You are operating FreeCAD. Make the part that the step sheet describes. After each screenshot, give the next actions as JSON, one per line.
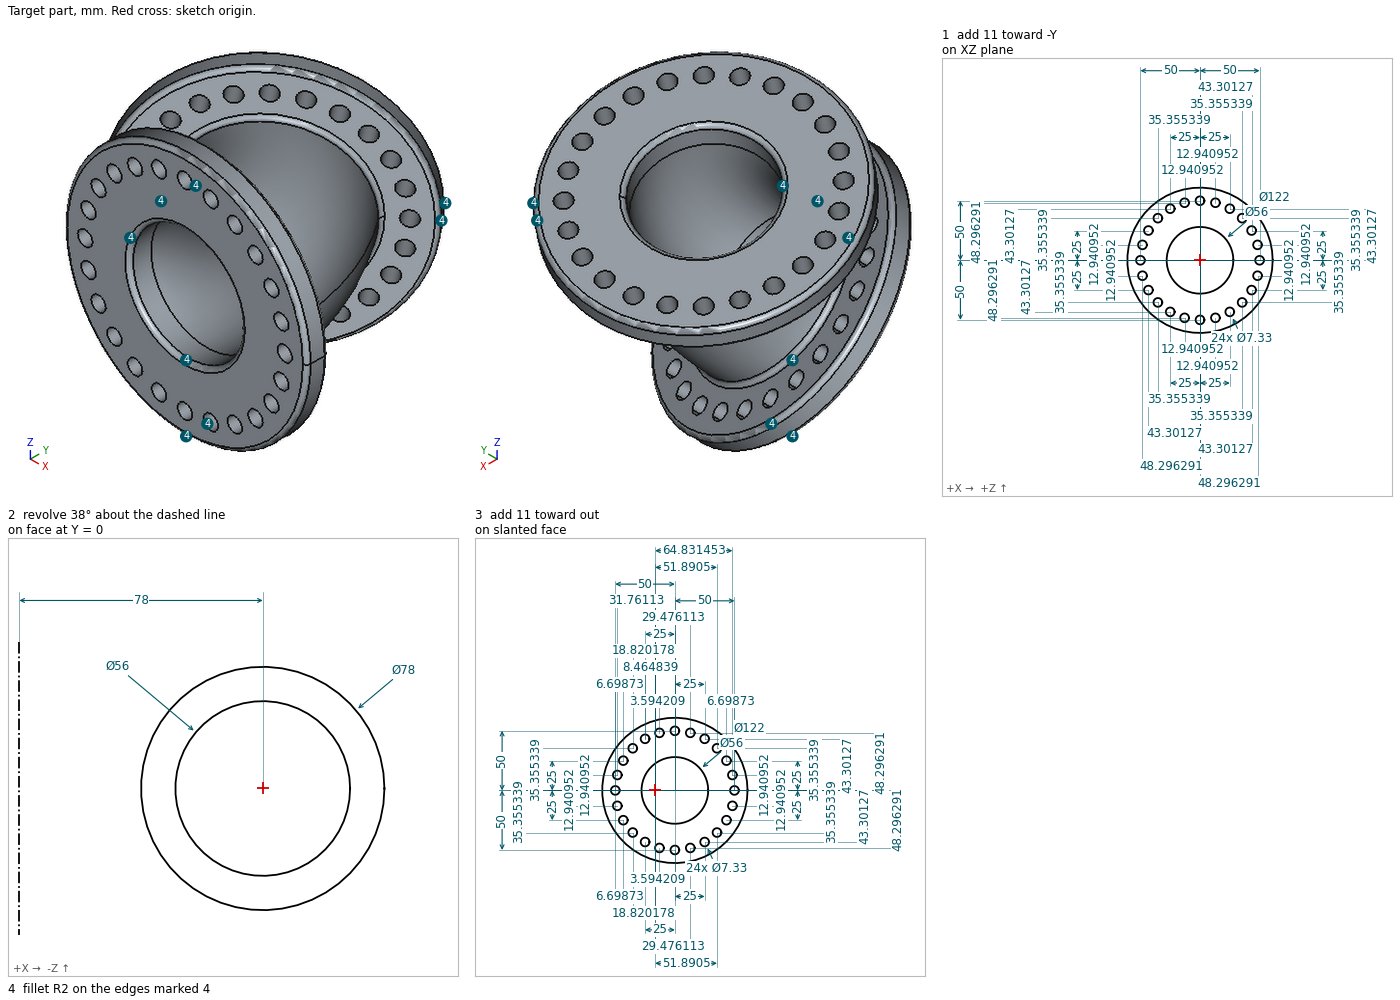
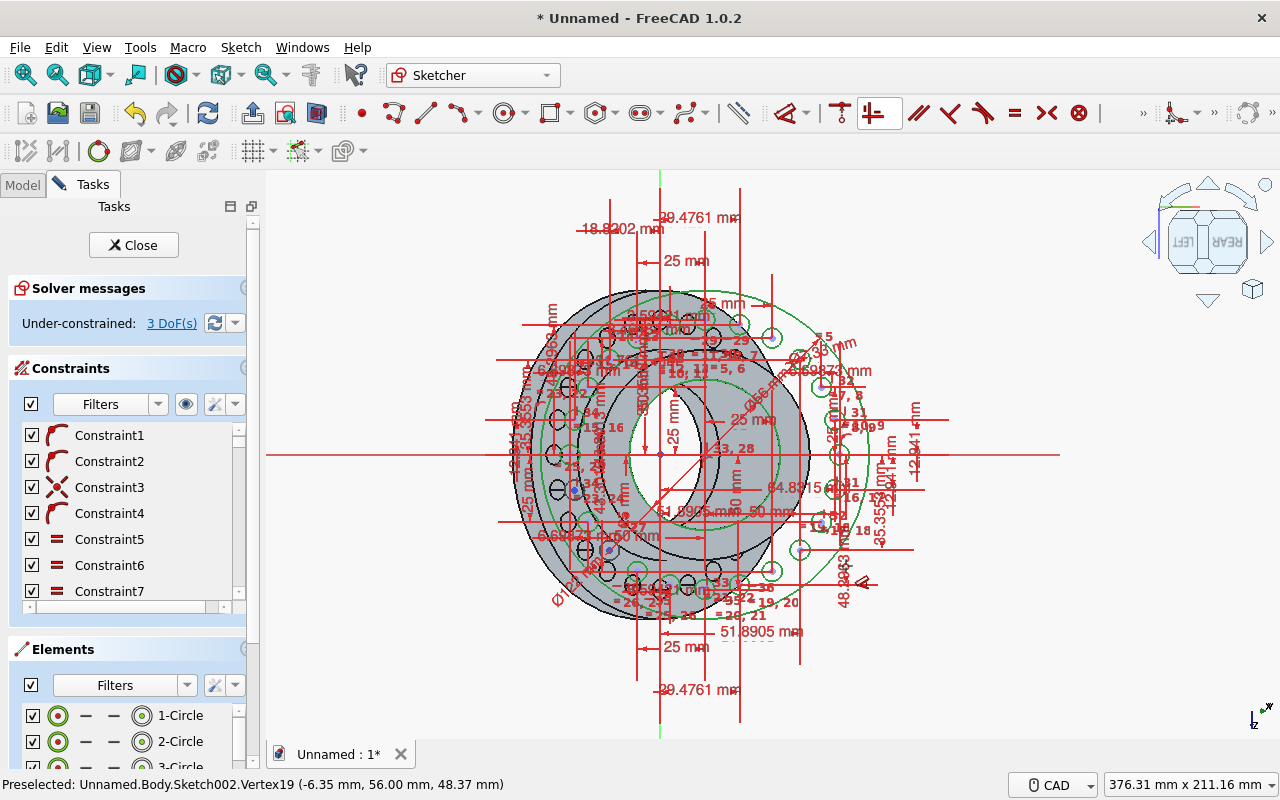
{"action": "left_click", "coordinate": [575, 490]}
{"action": "left_click", "coordinate": [445, 472]}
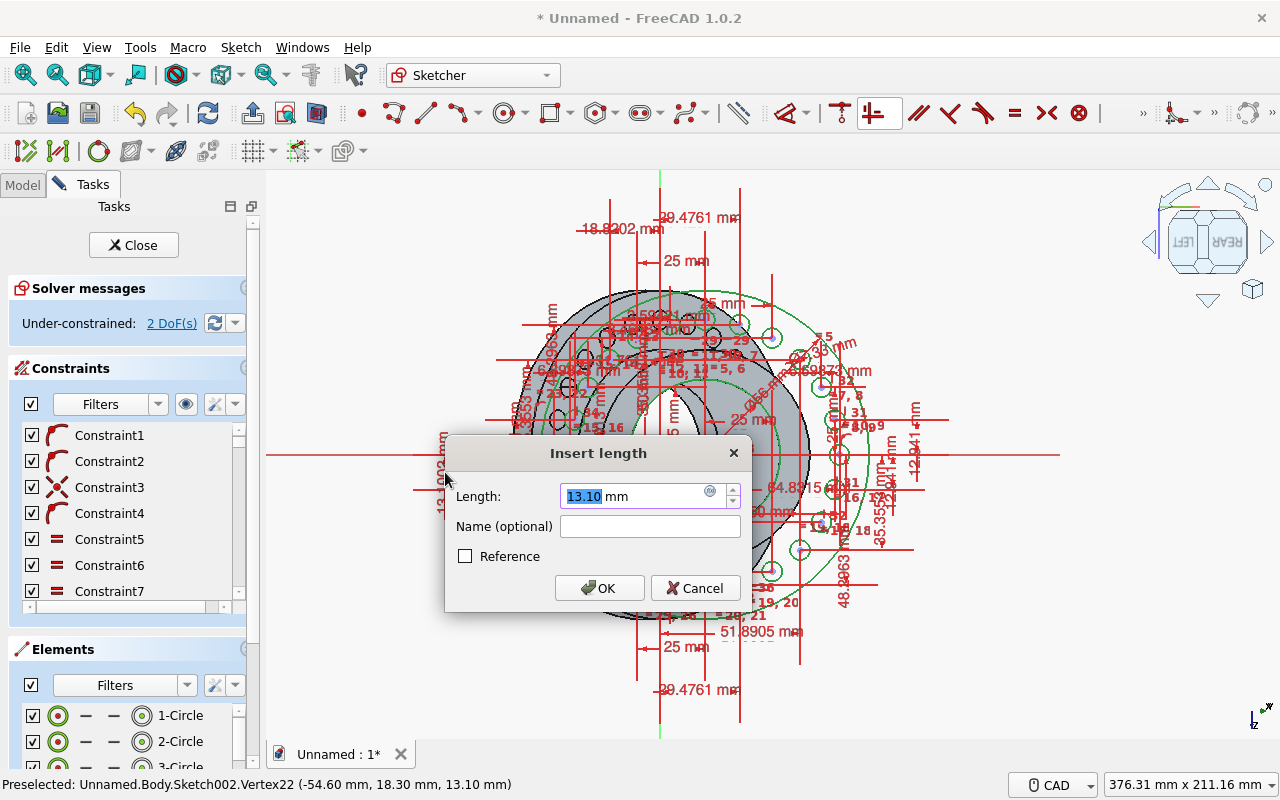
{"action": "type", "text": "12.940952"}
{"action": "key", "text": "Return"}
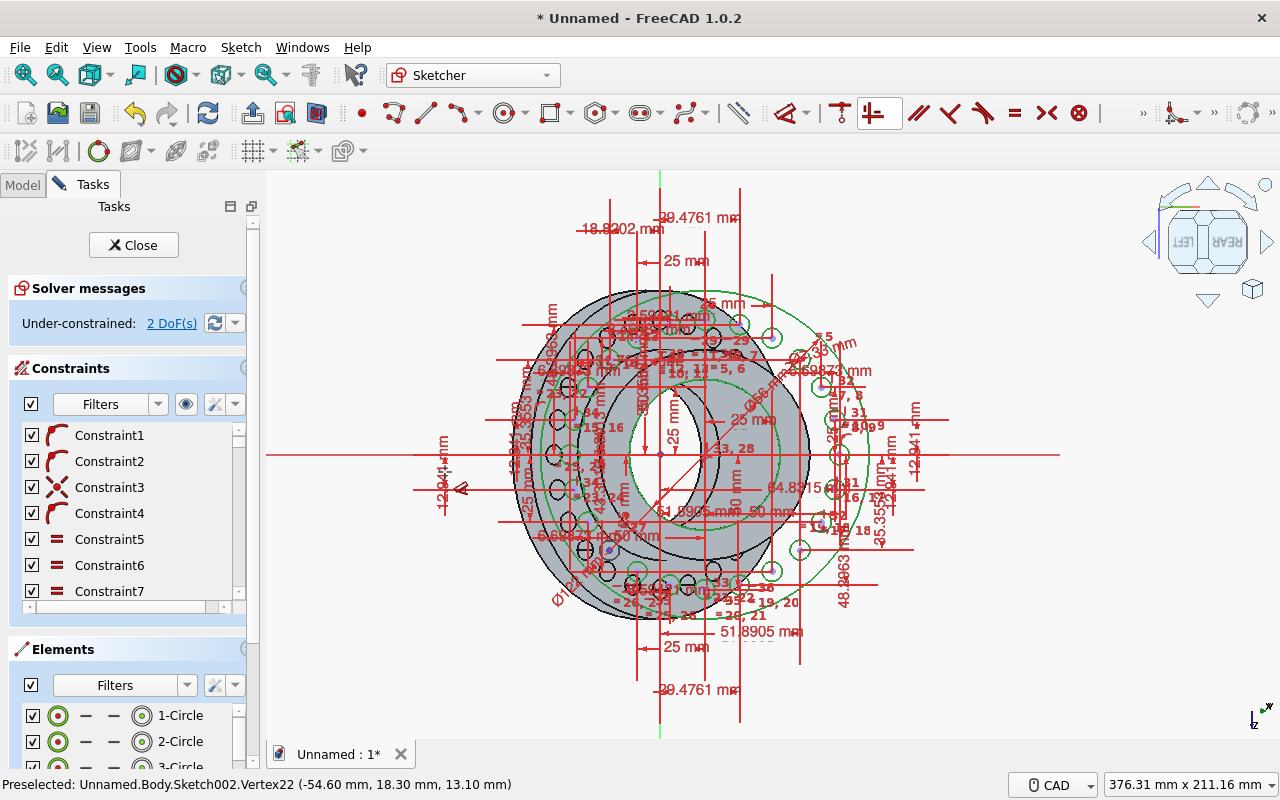
{"action": "left_click", "coordinate": [610, 550]}
{"action": "left_click", "coordinate": [623, 680]}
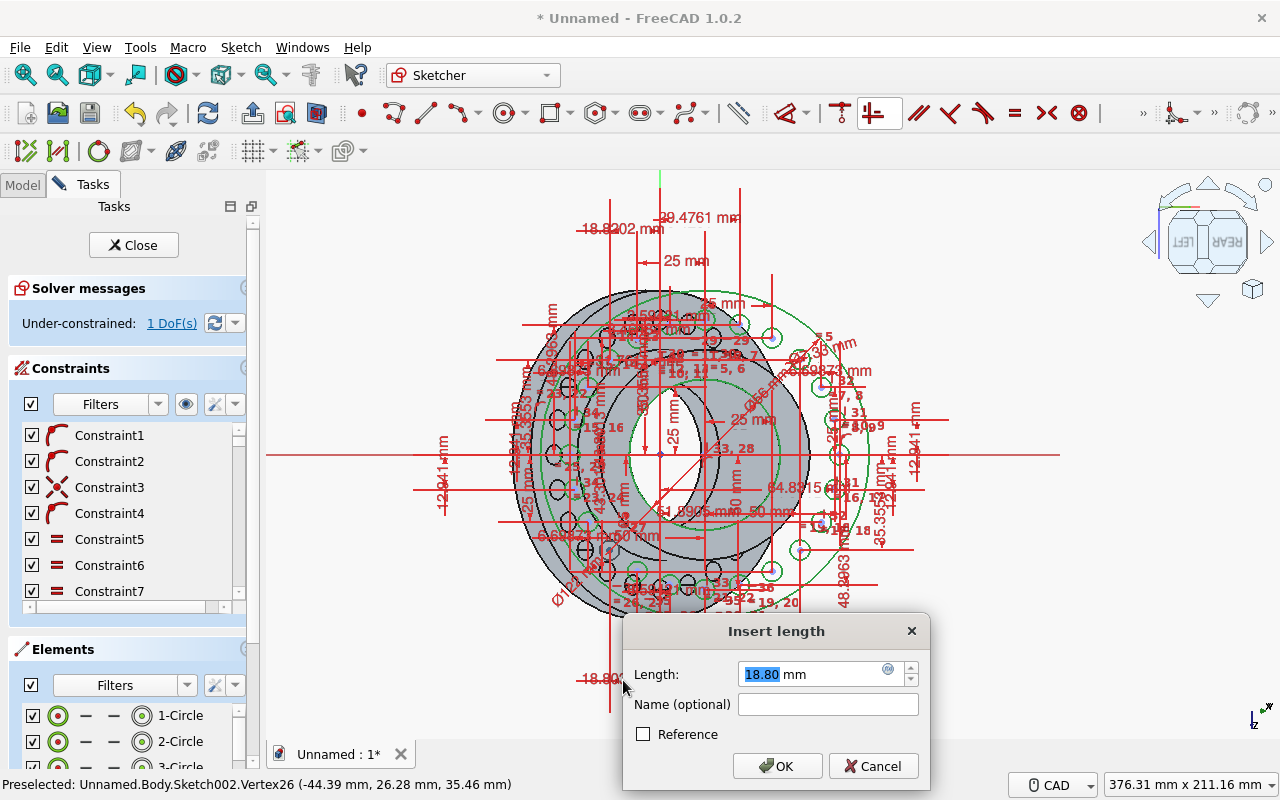
{"action": "type", "text": "18.820178"}
{"action": "key", "text": "Return"}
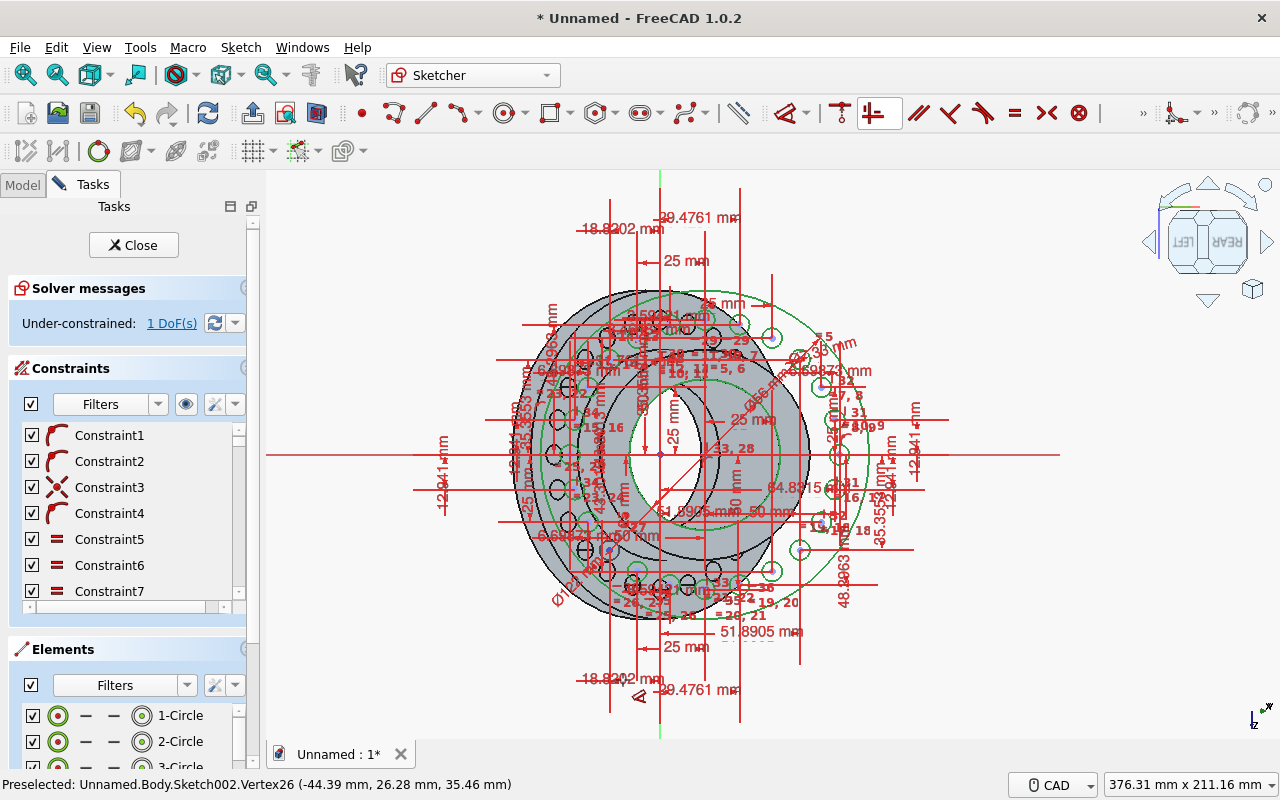
{"action": "left_click", "coordinate": [610, 550]}
{"action": "left_click", "coordinate": [694, 469]}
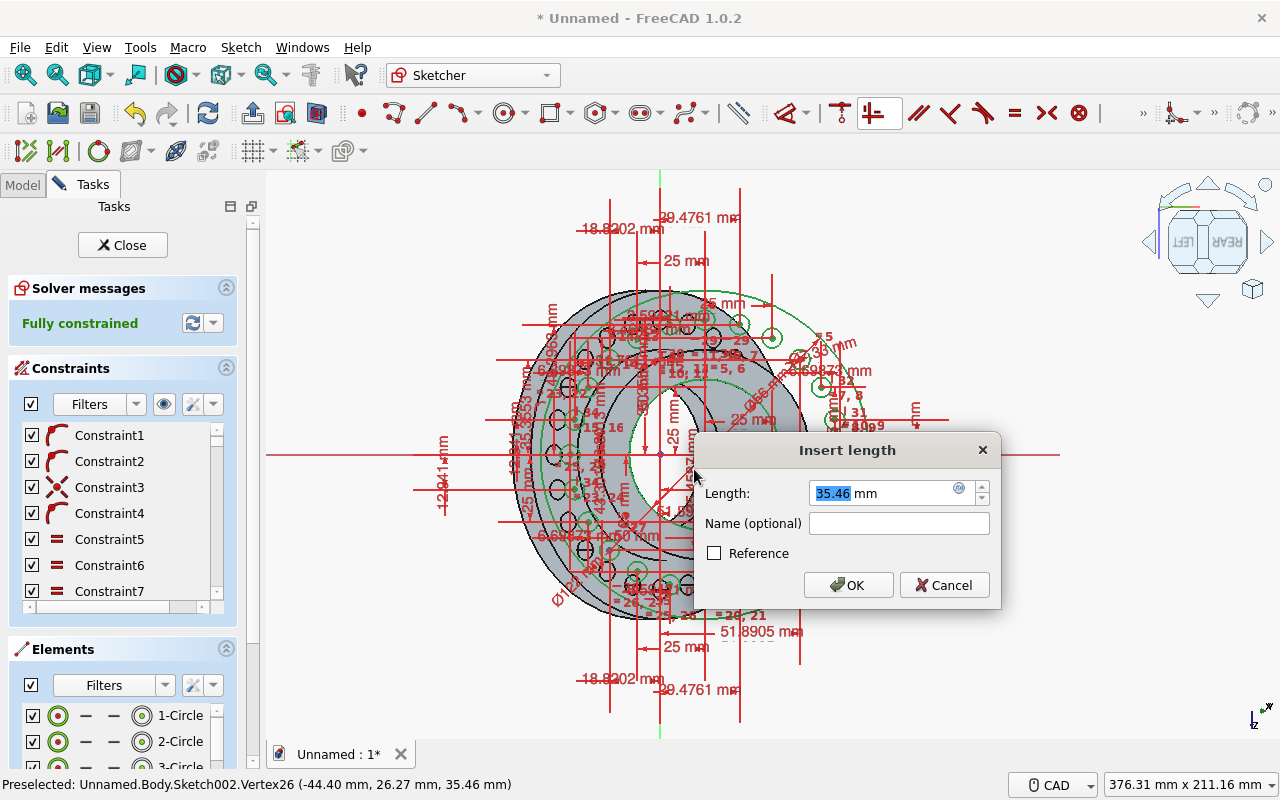
{"action": "type", "text": "35.355339"}
{"action": "key", "text": "Return"}
{"action": "key", "text": "Escape"}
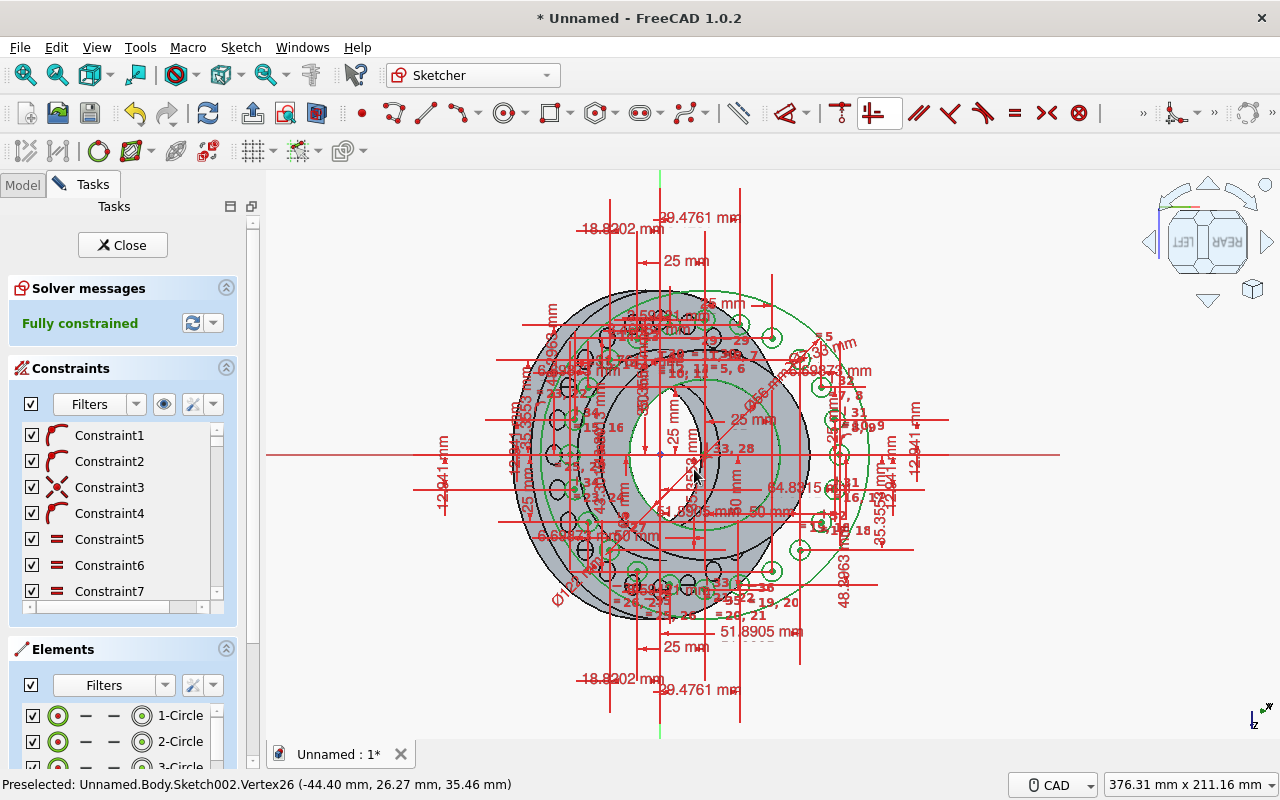
{"action": "left_click", "coordinate": [123, 245]}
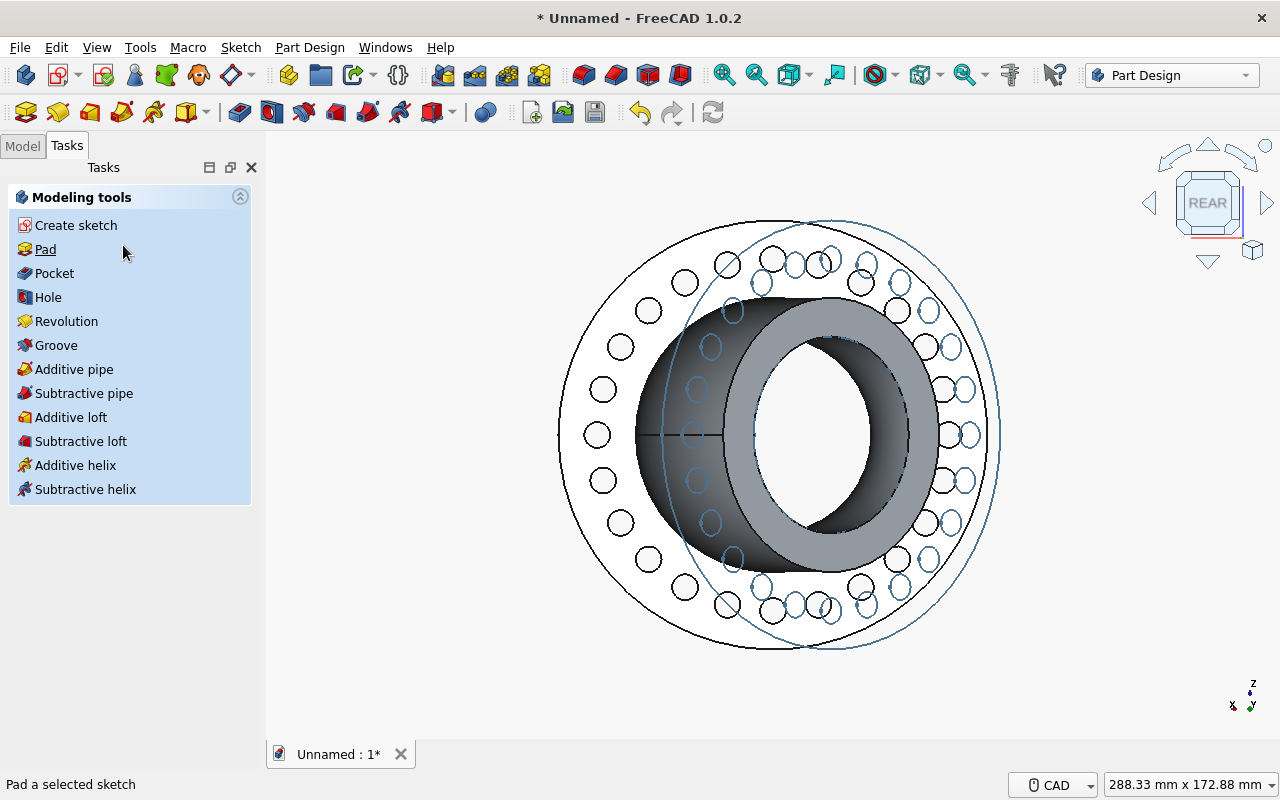
{"action": "left_click", "coordinate": [26, 112]}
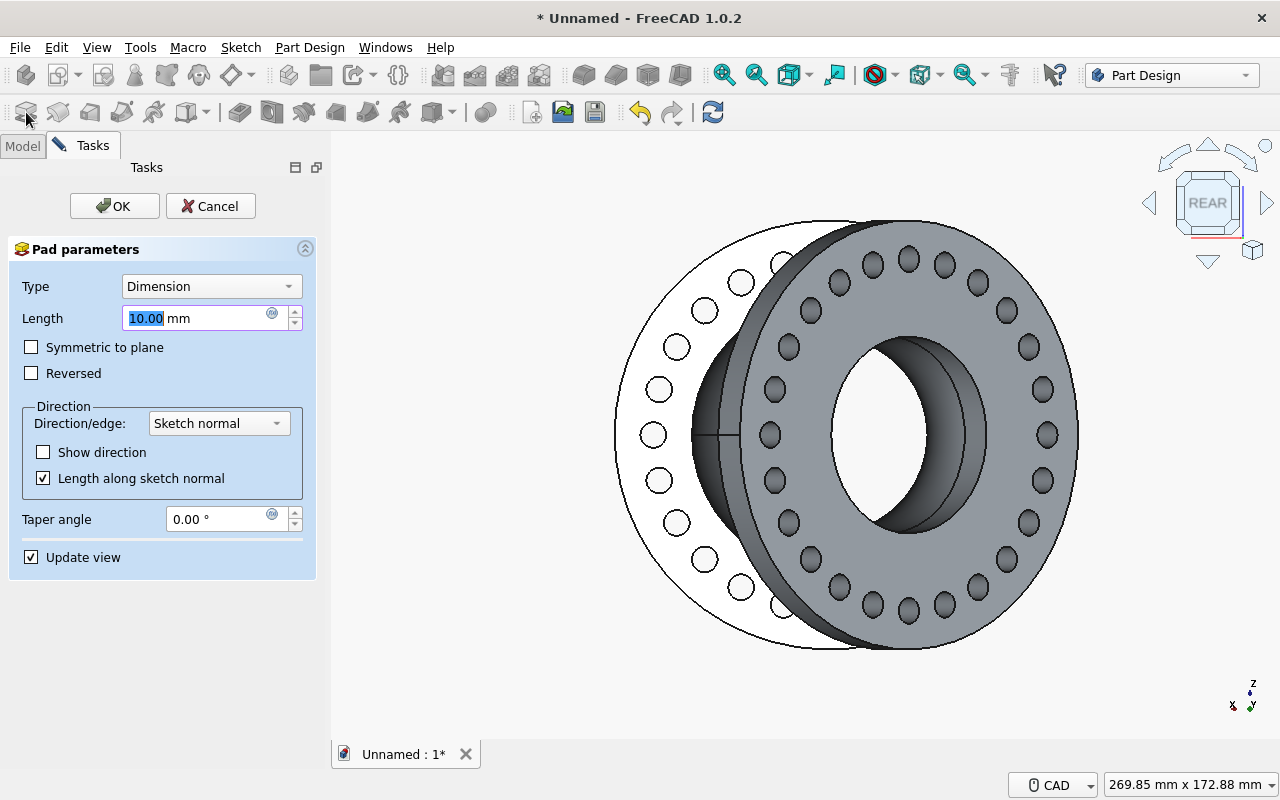
{"action": "type", "text": "11"}
{"action": "key", "text": "Tab"}